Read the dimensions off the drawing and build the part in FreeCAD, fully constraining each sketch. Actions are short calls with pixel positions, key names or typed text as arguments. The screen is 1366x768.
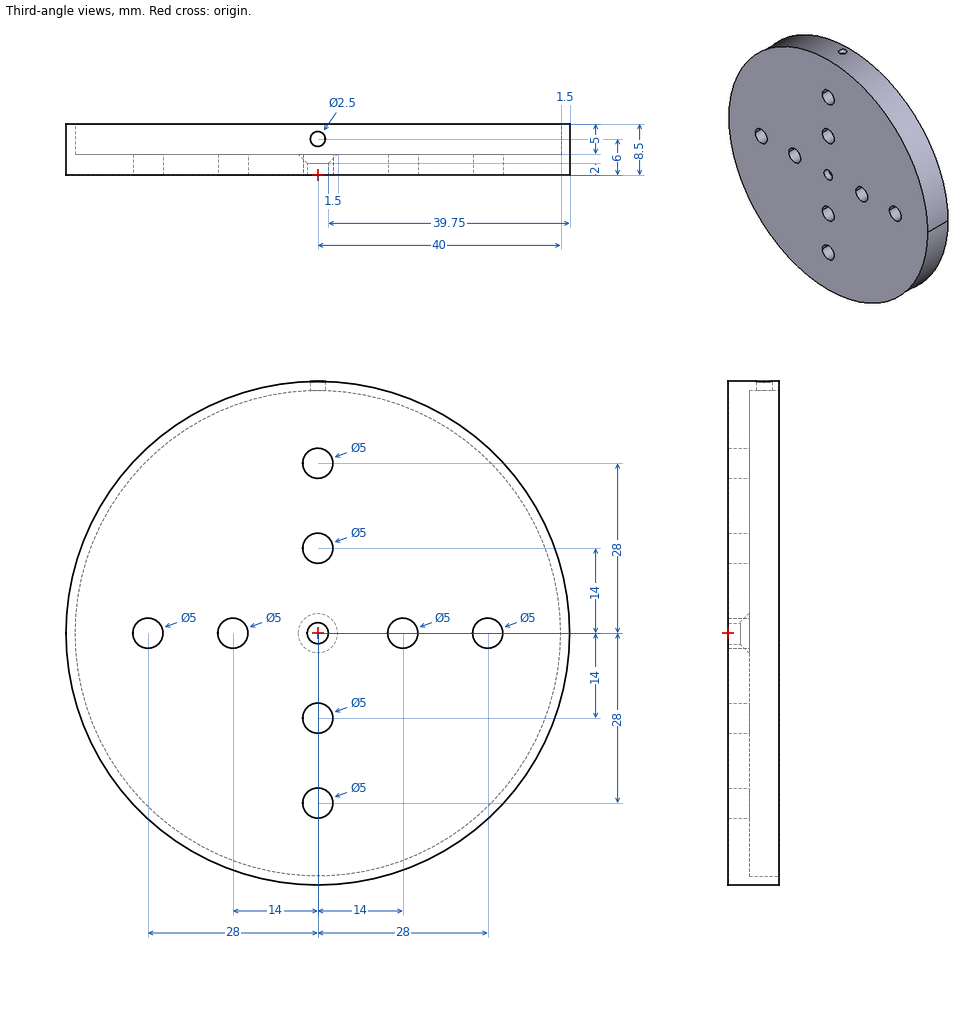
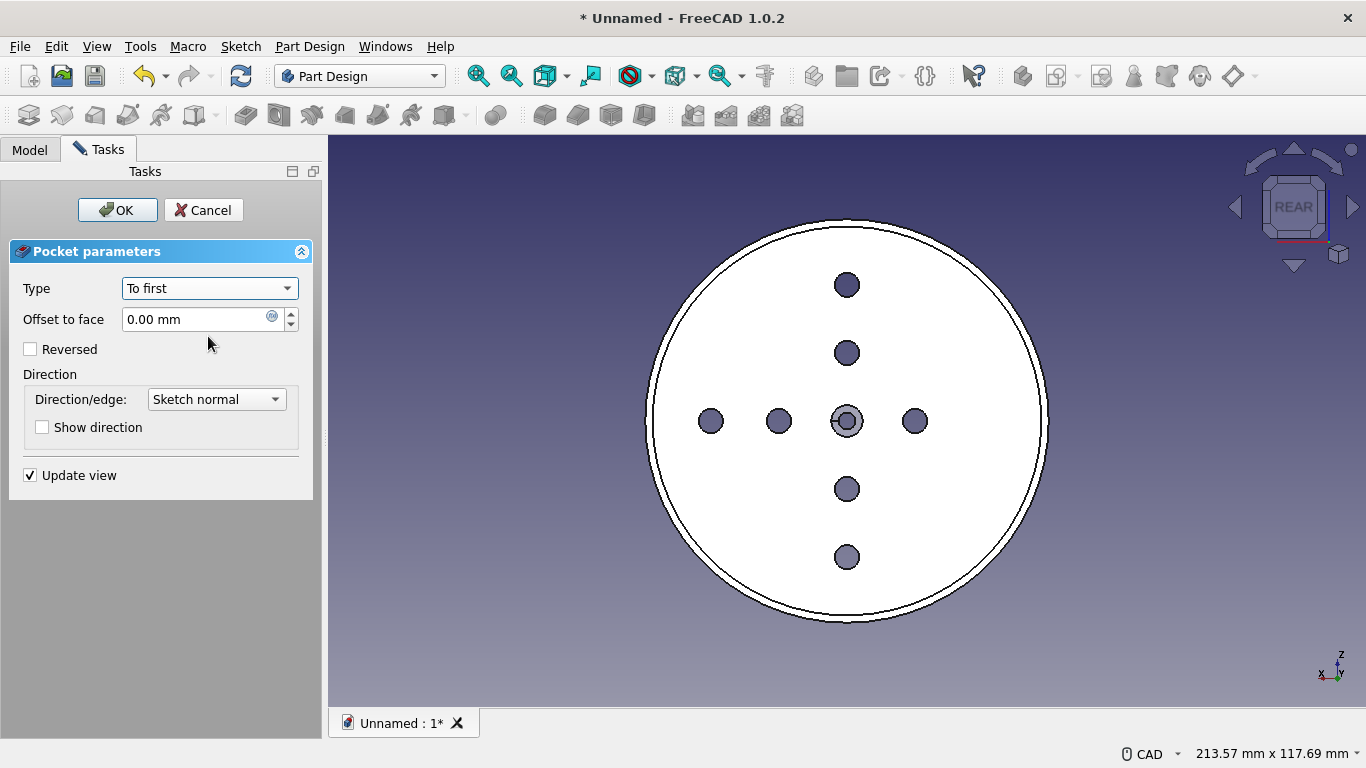
click(118, 210)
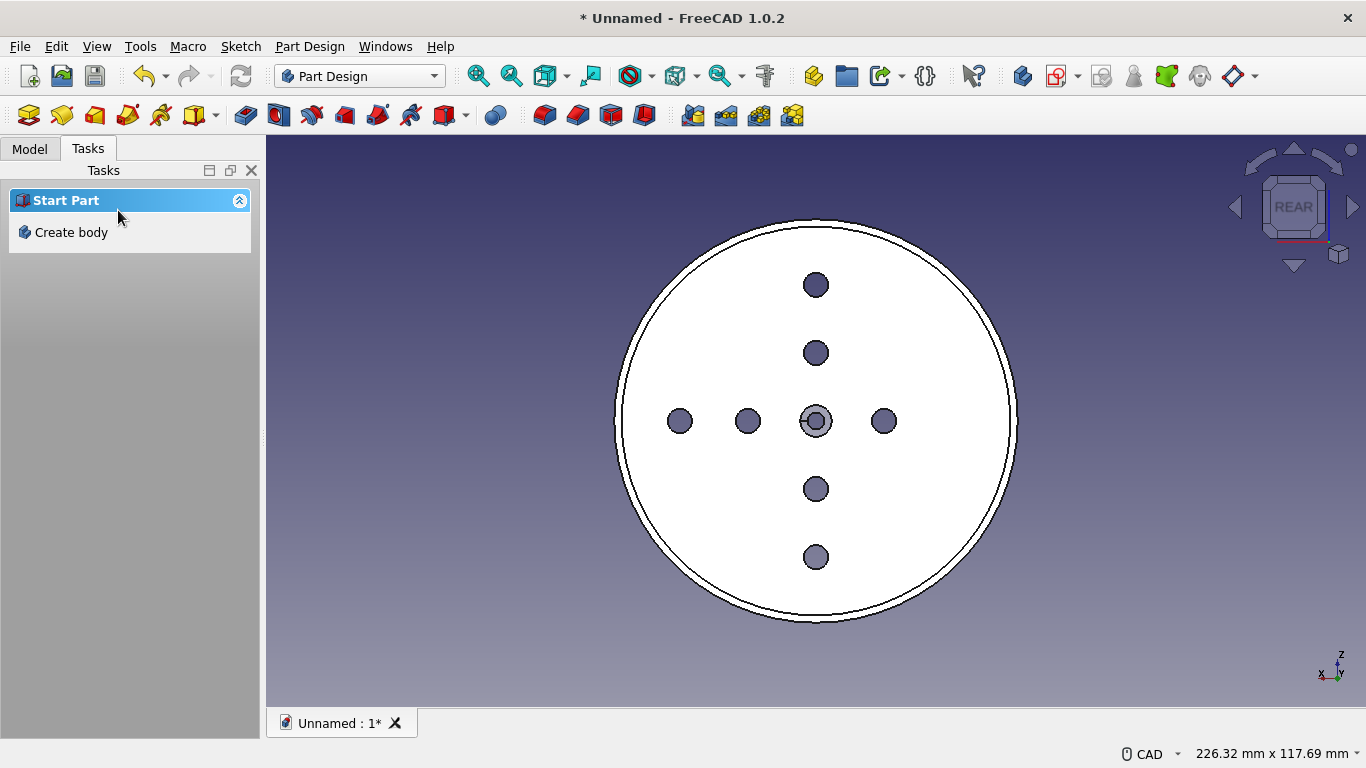
click(927, 364)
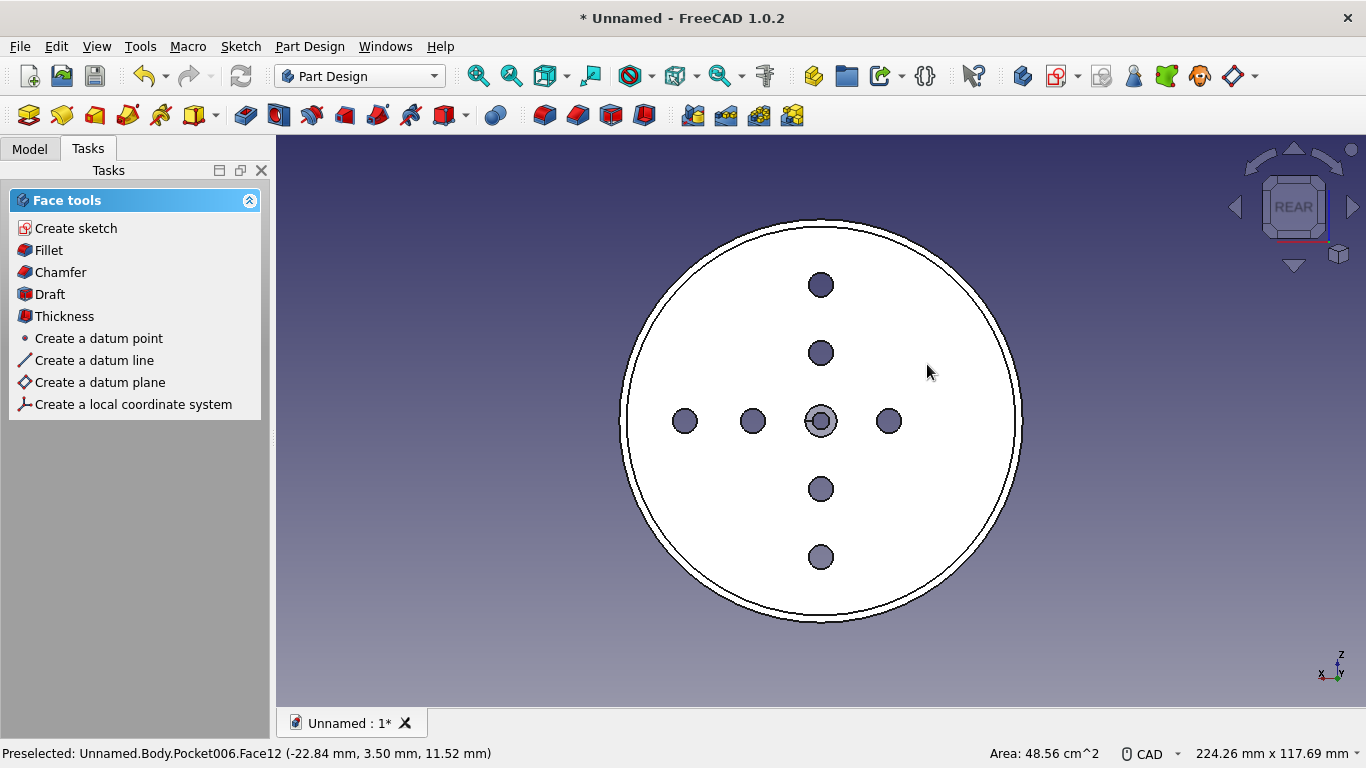
click(1056, 76)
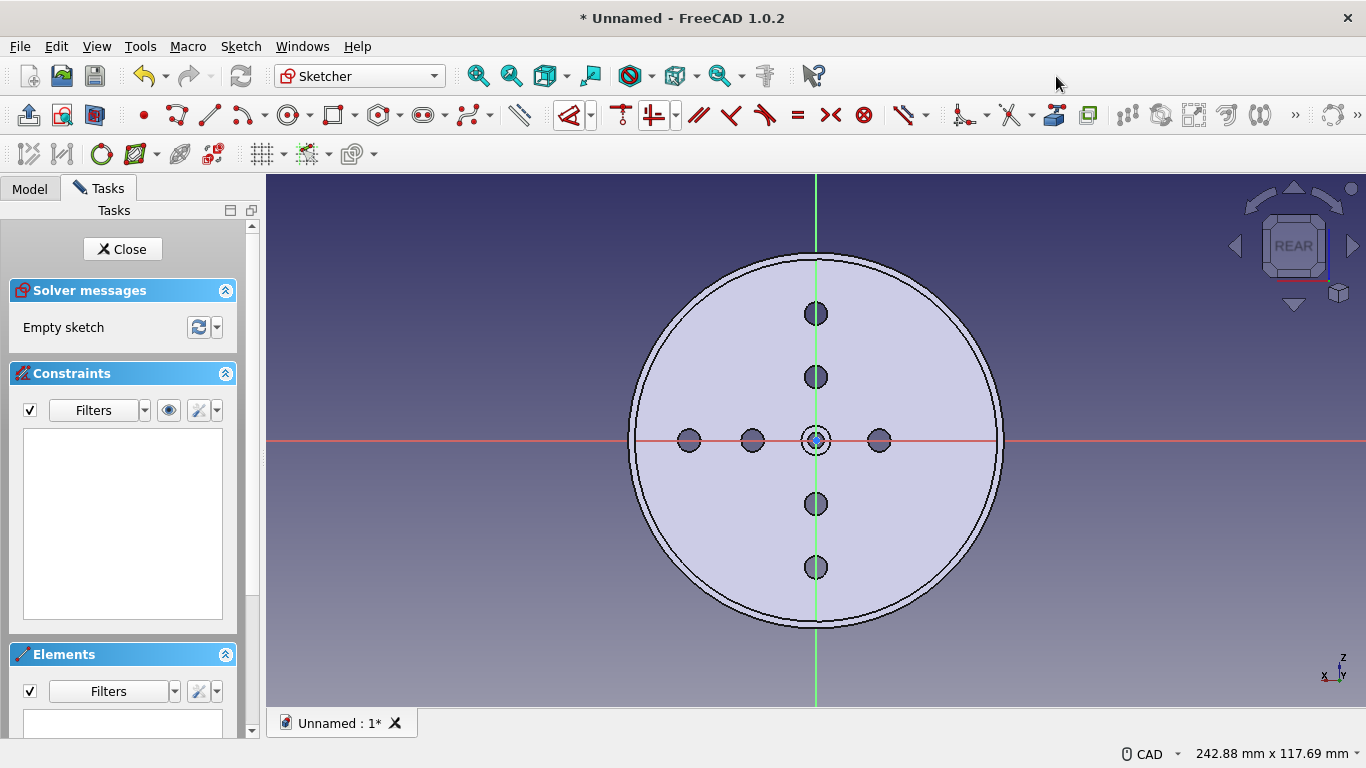
scroll(958, 441, up, 13)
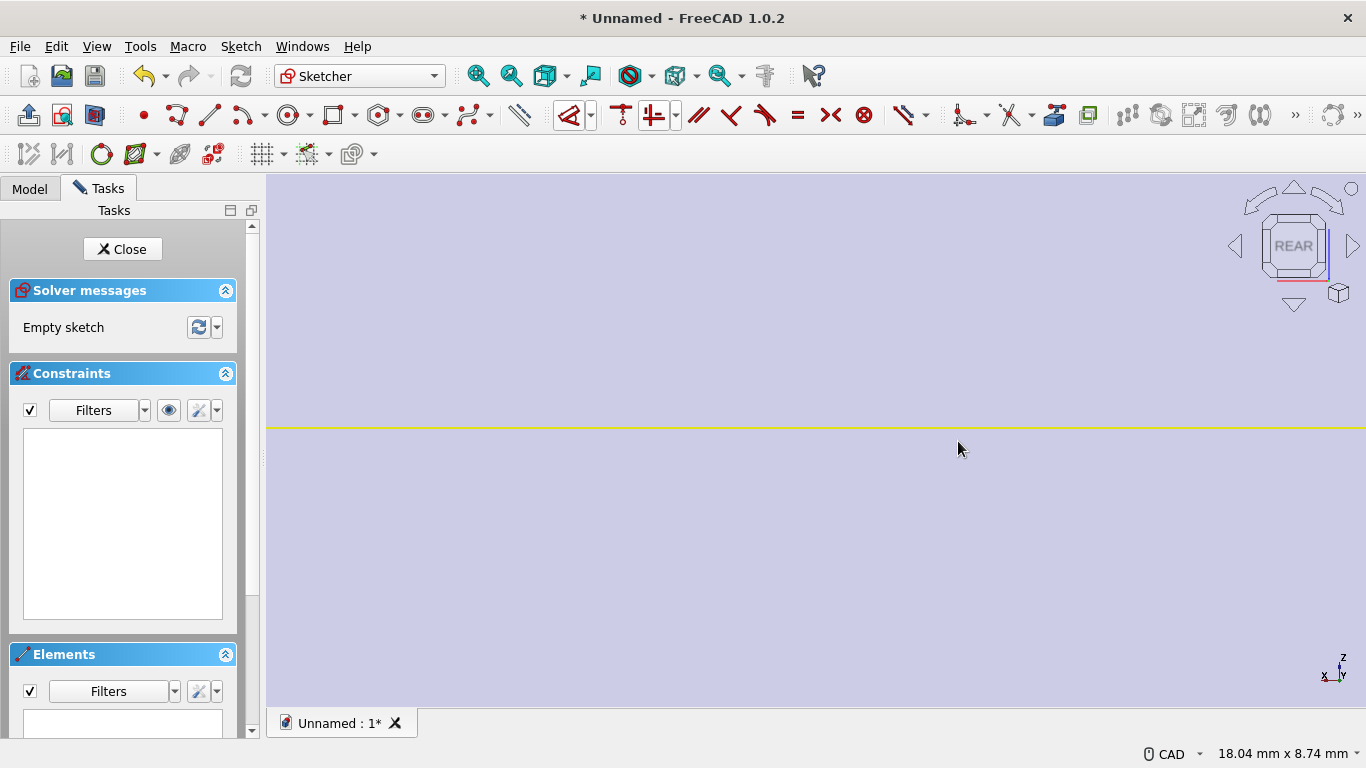
click(288, 116)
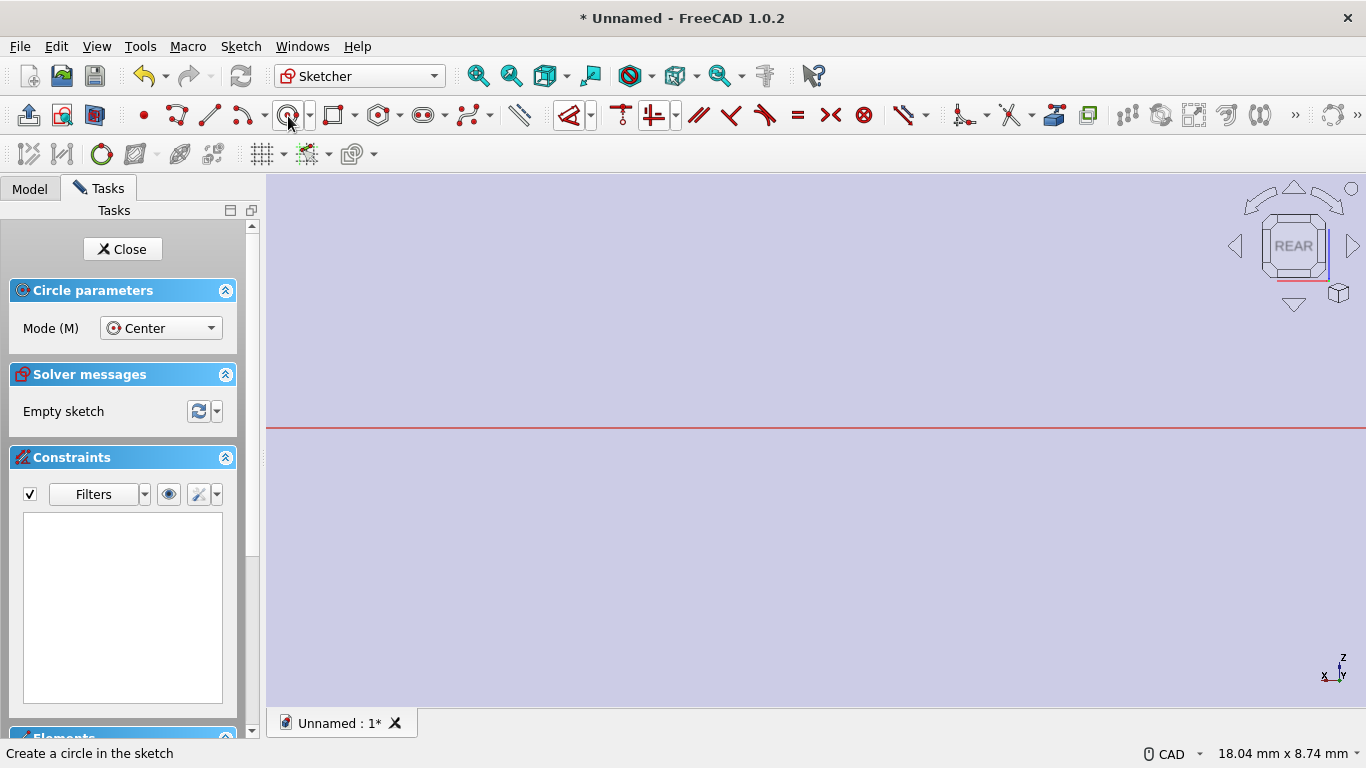
click(746, 428)
click(853, 320)
key(Escape)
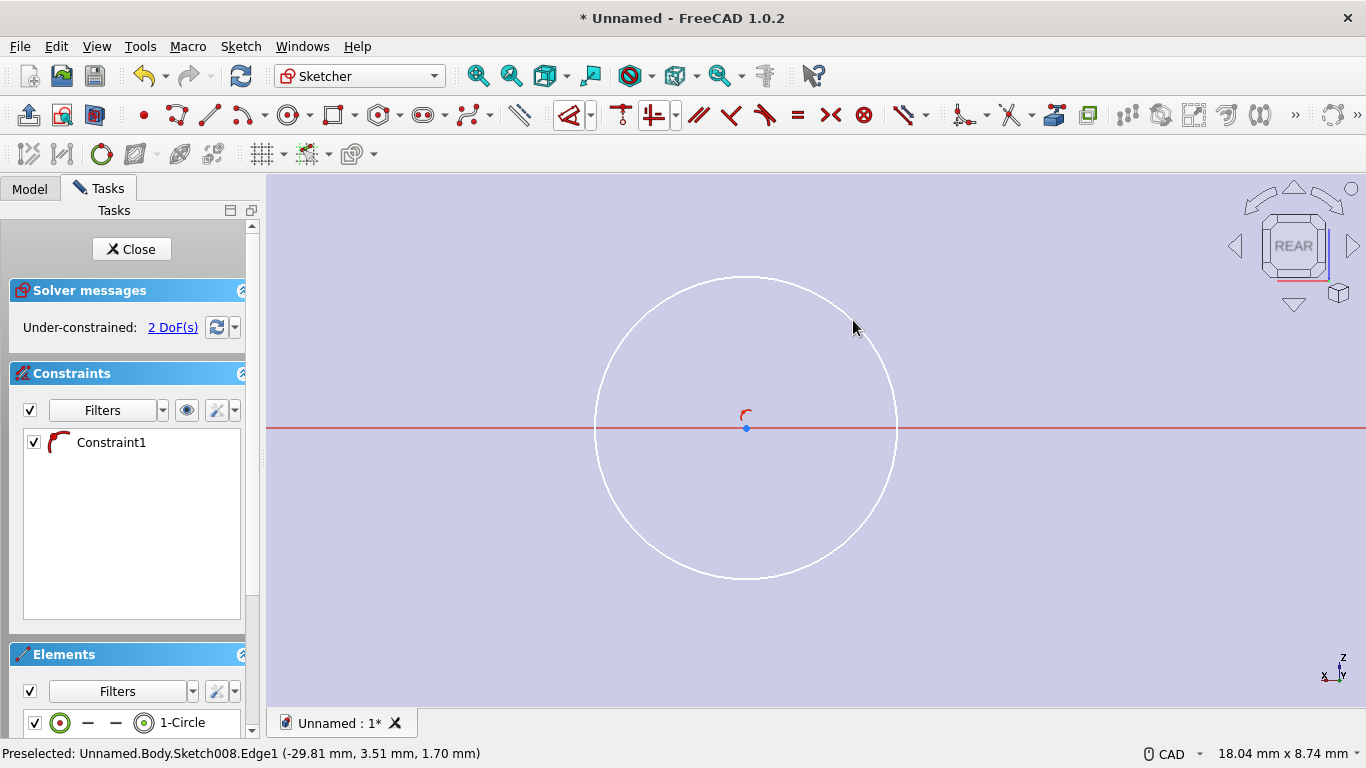
click(853, 321)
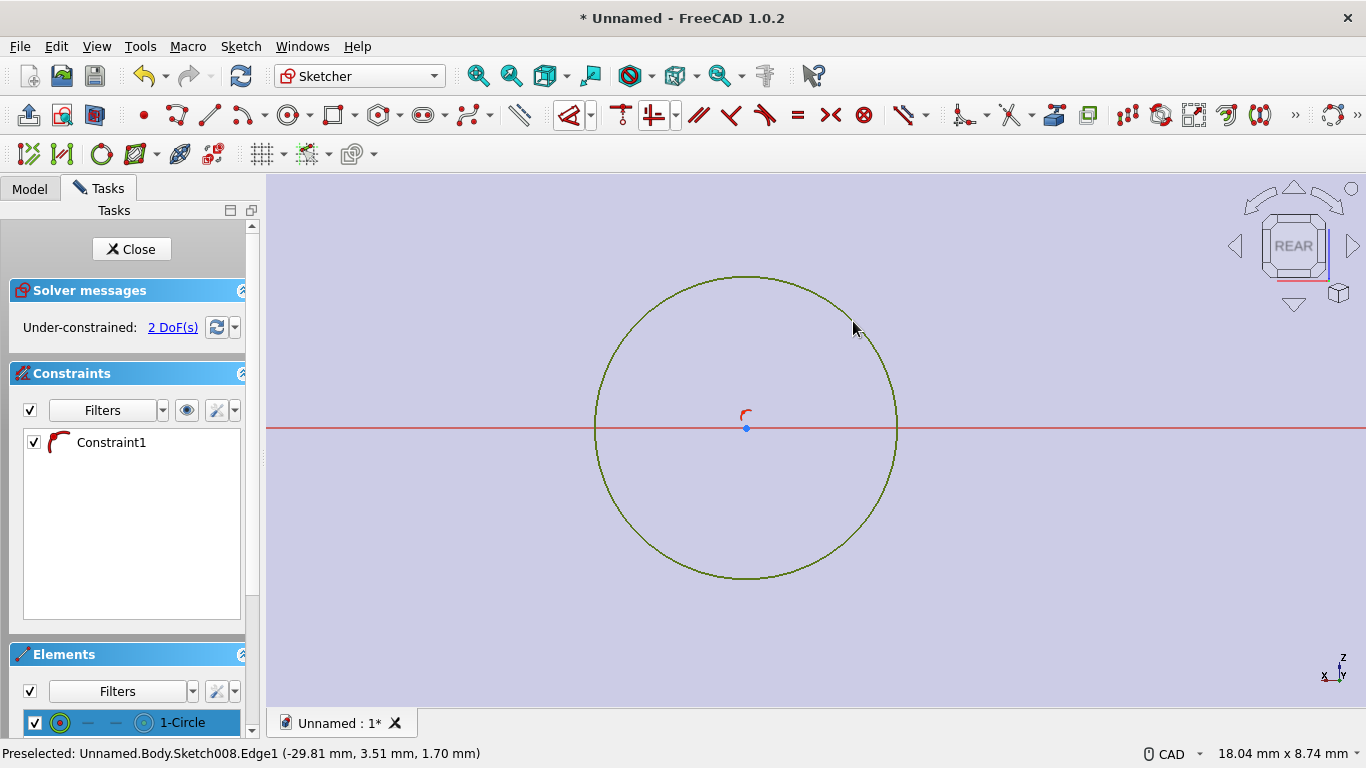
click(590, 116)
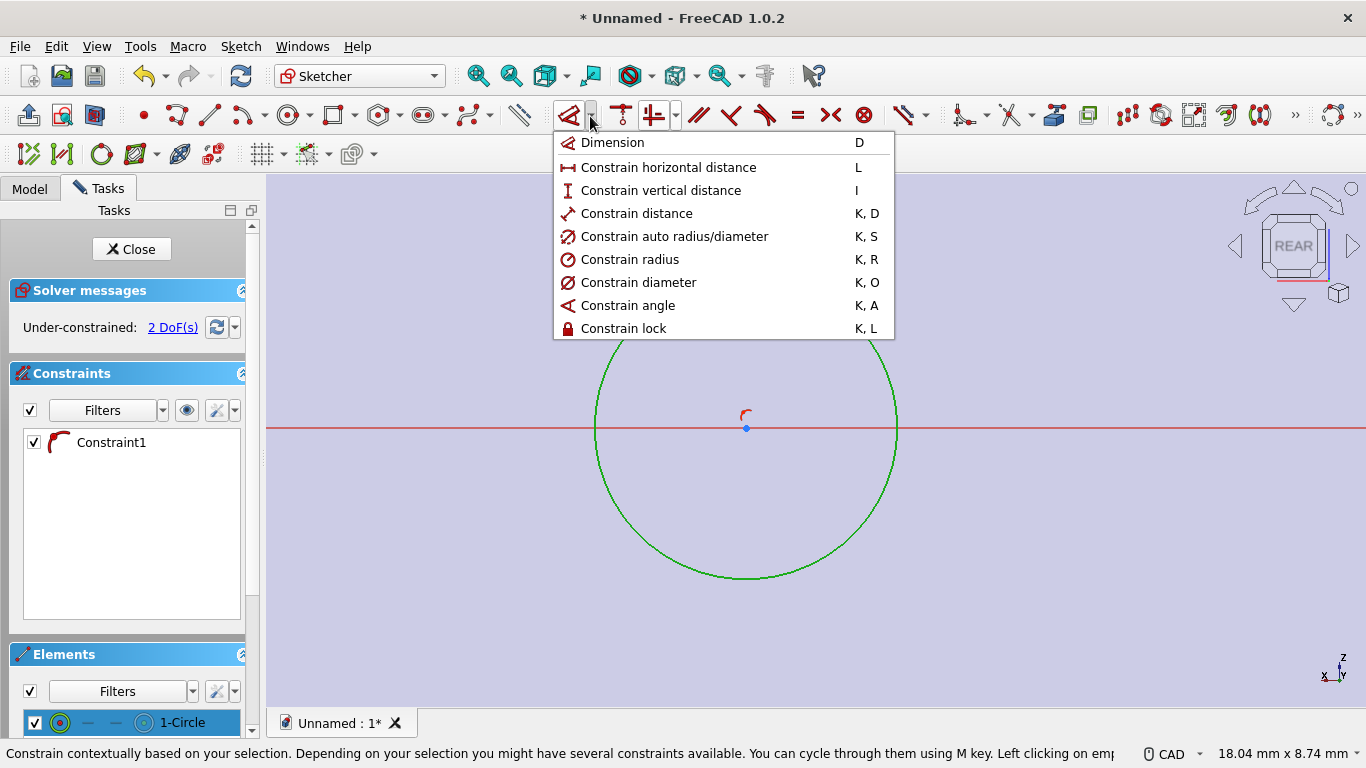
click(724, 282)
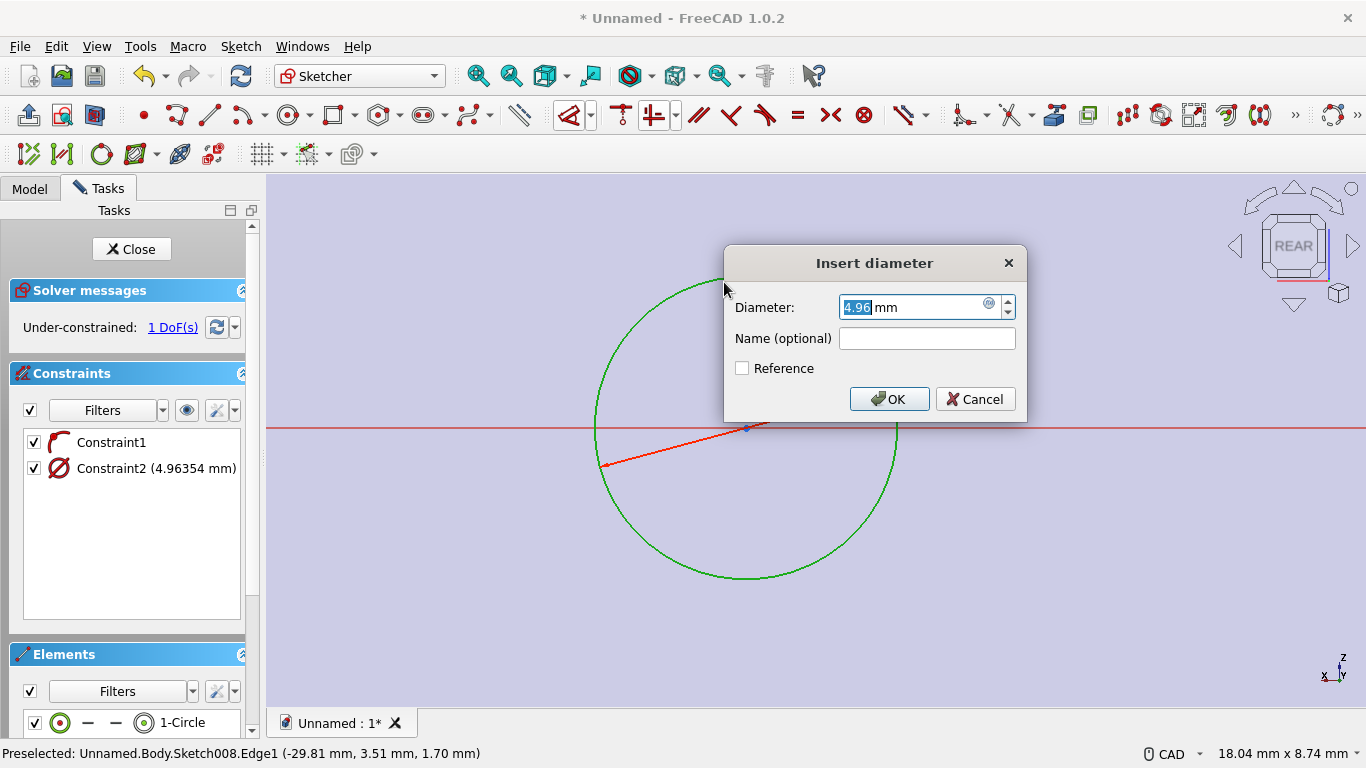
text(5)
key(Return)